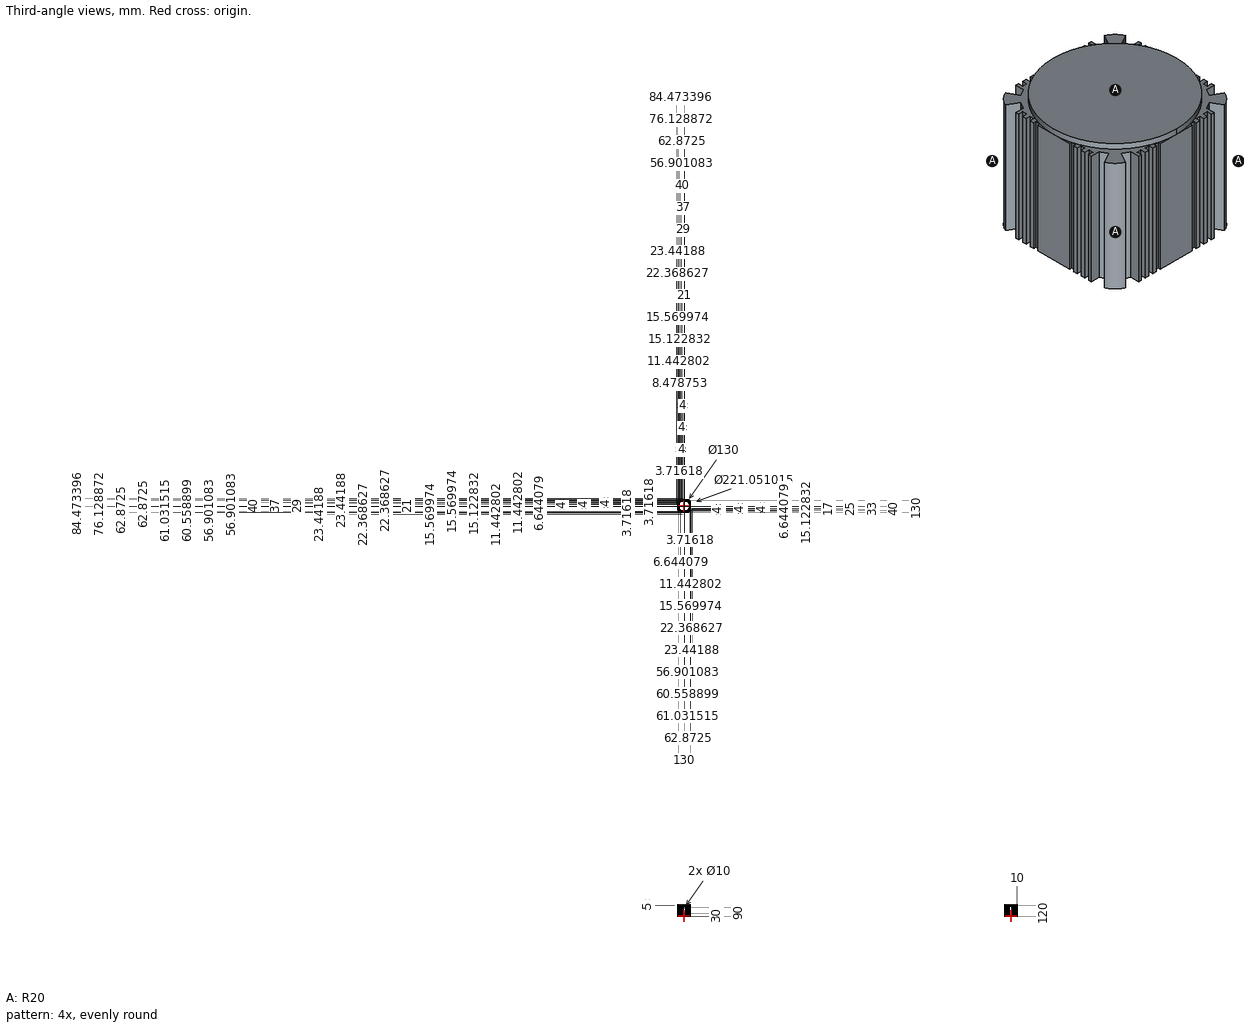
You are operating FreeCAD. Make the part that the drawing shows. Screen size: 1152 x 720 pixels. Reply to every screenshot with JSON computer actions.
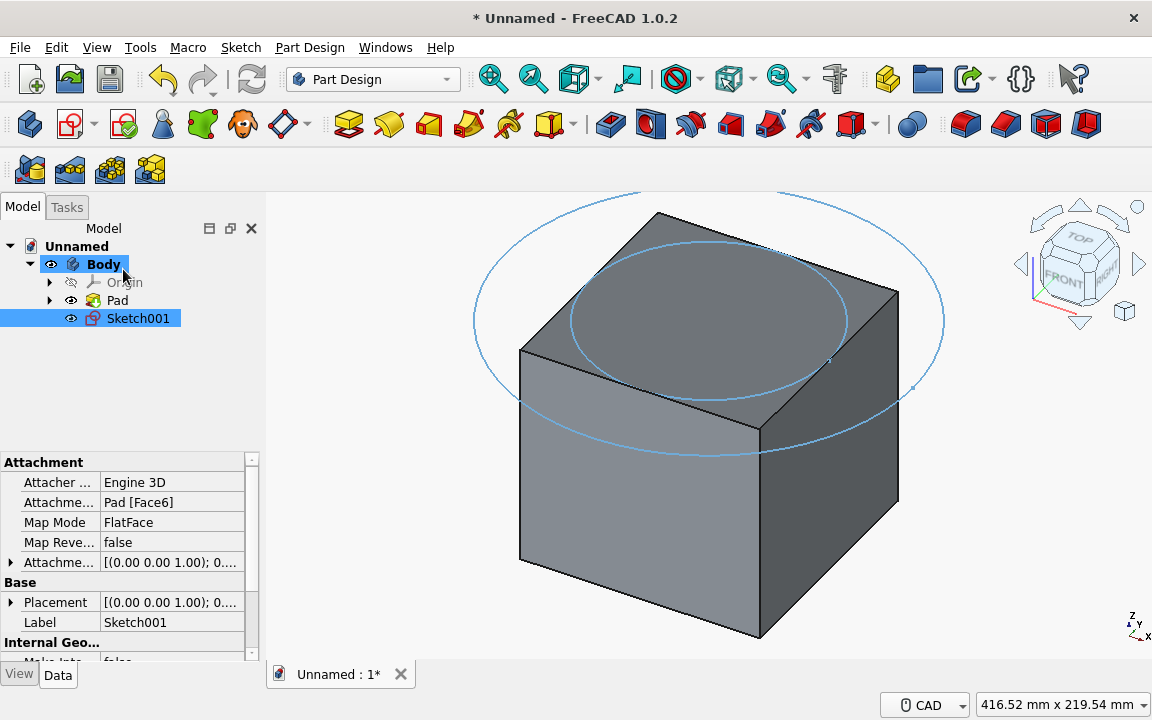
{"action": "left_click", "coordinate": [612, 124]}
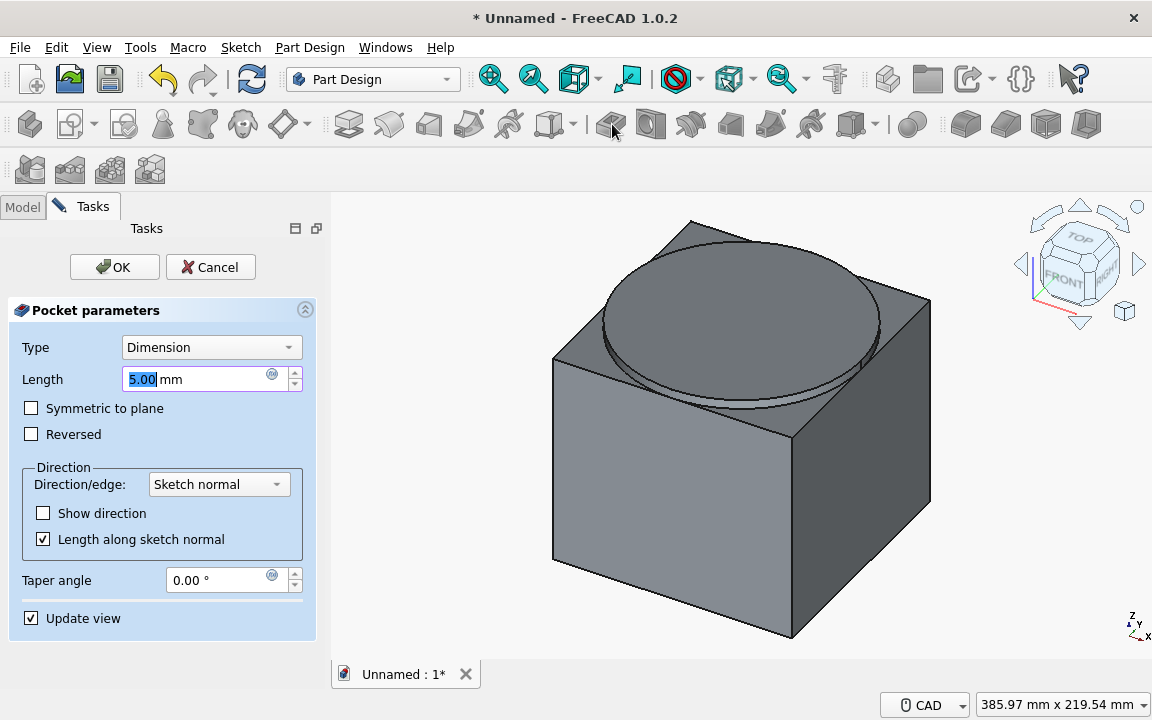
{"action": "type", "text": "5"}
{"action": "key", "text": "Tab"}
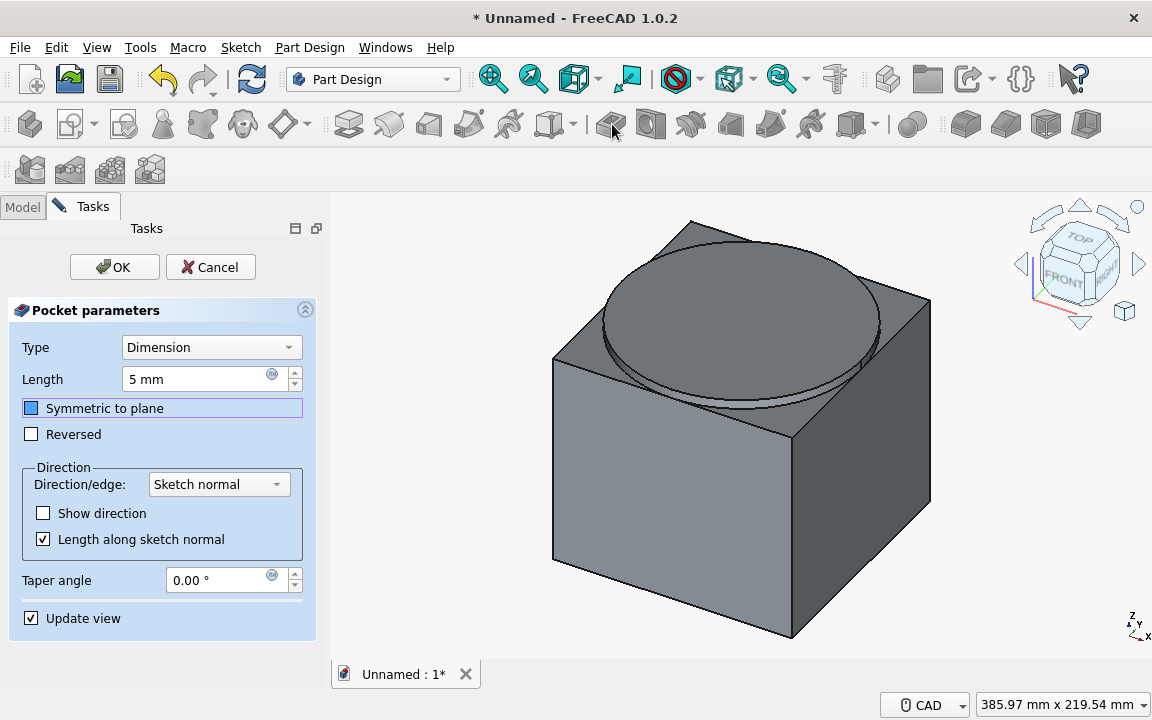
{"action": "left_click", "coordinate": [115, 267]}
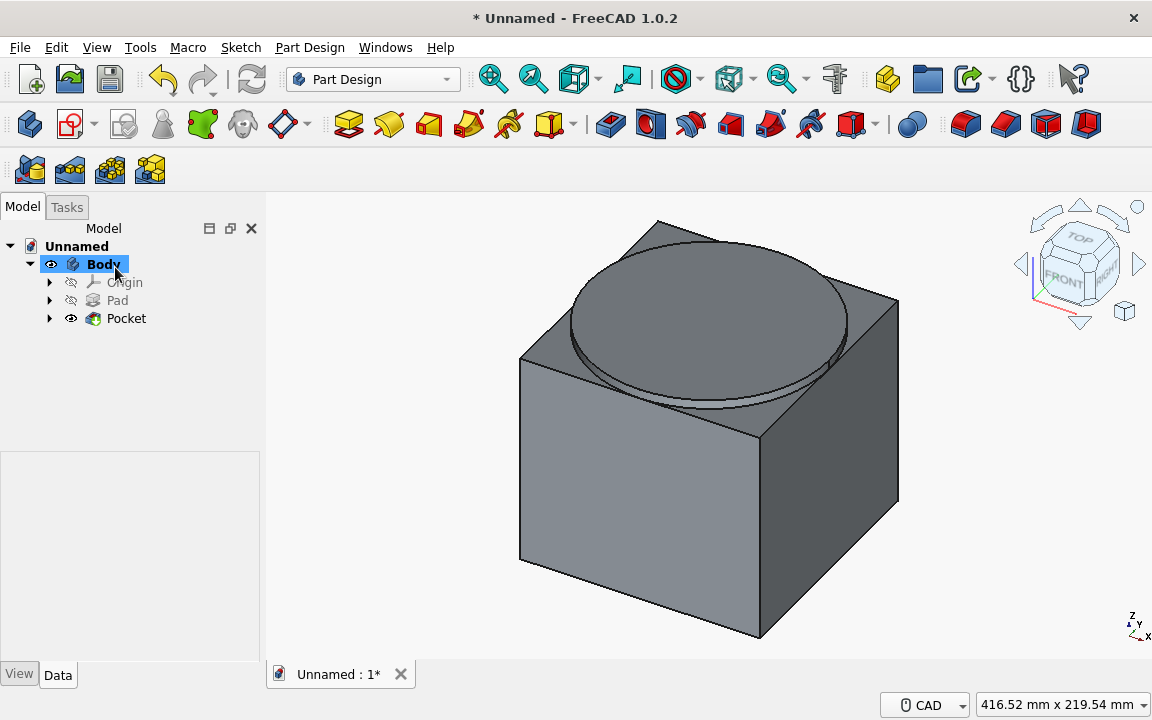
{"action": "left_click", "coordinate": [760, 537]}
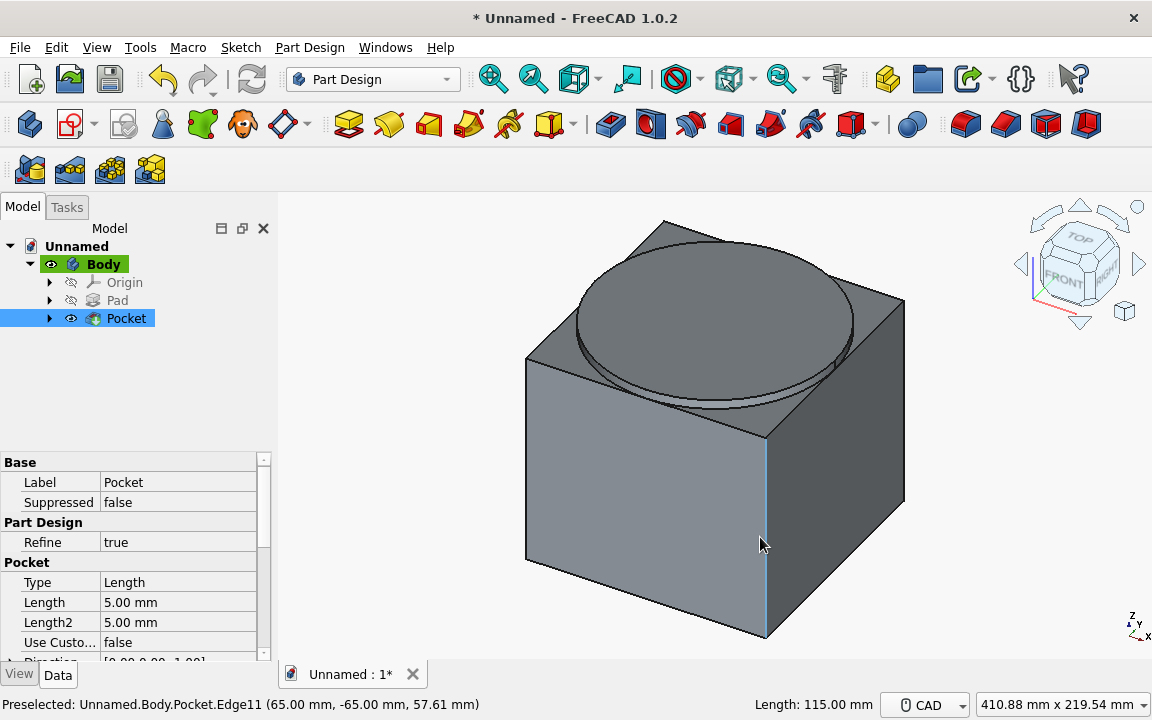
{"action": "key", "text": "0"}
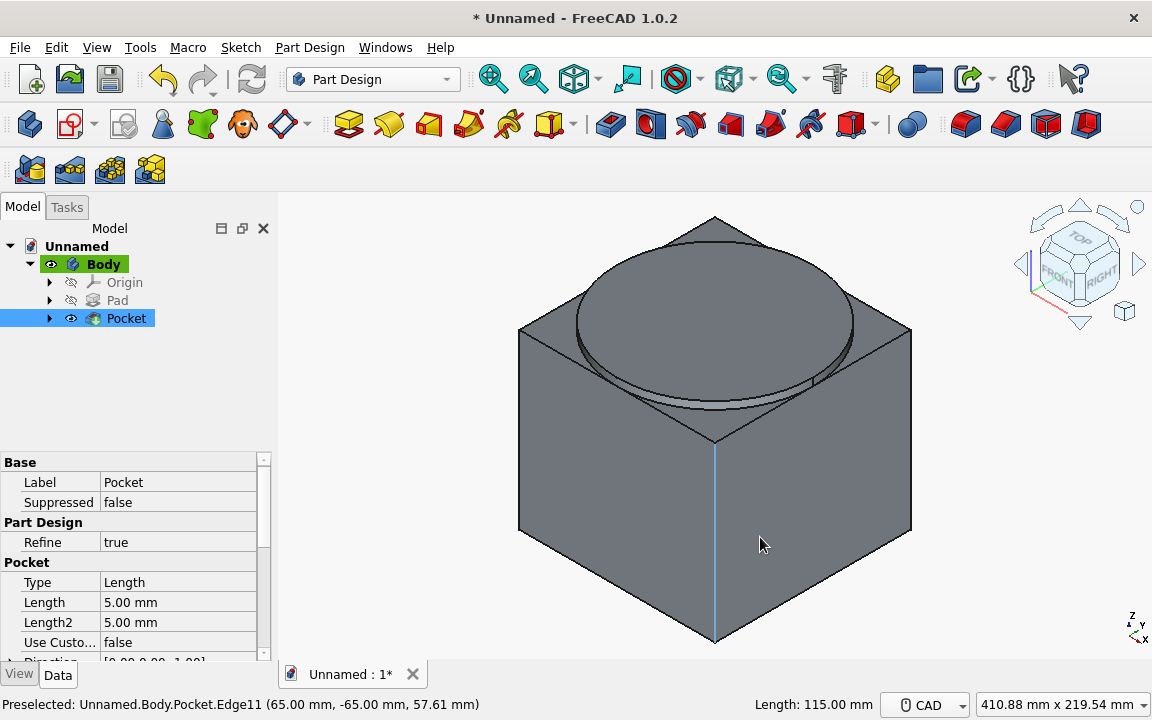
{"action": "key", "text": "2"}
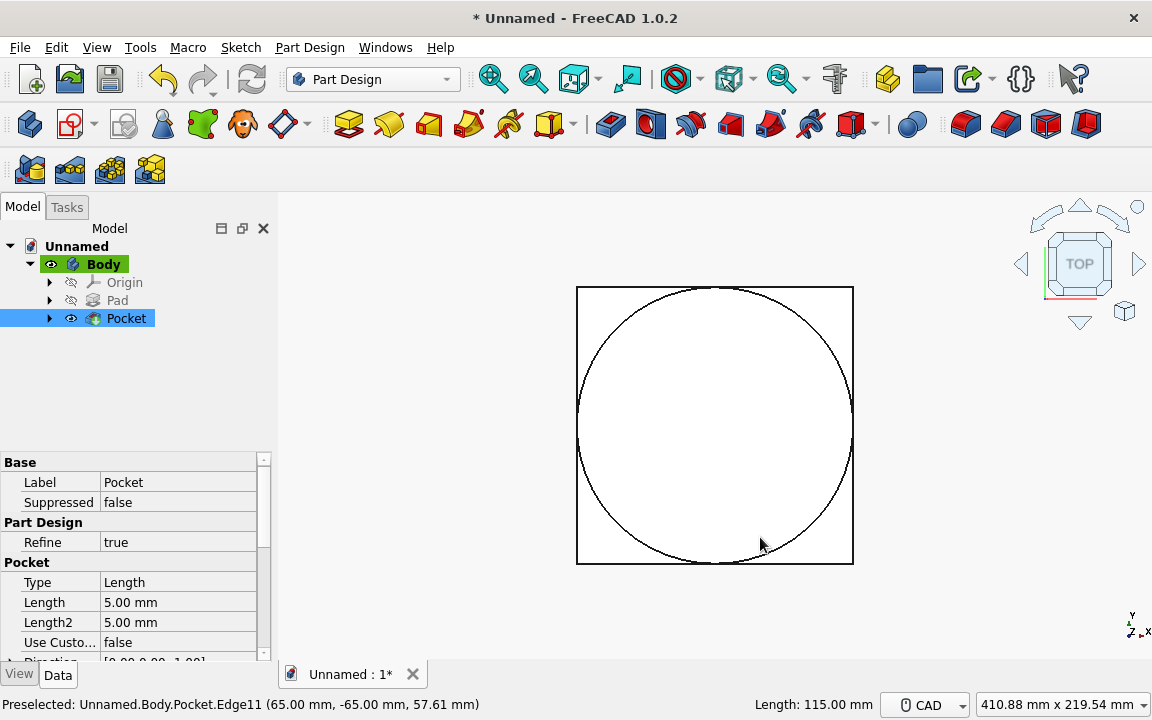
{"action": "key", "text": "1"}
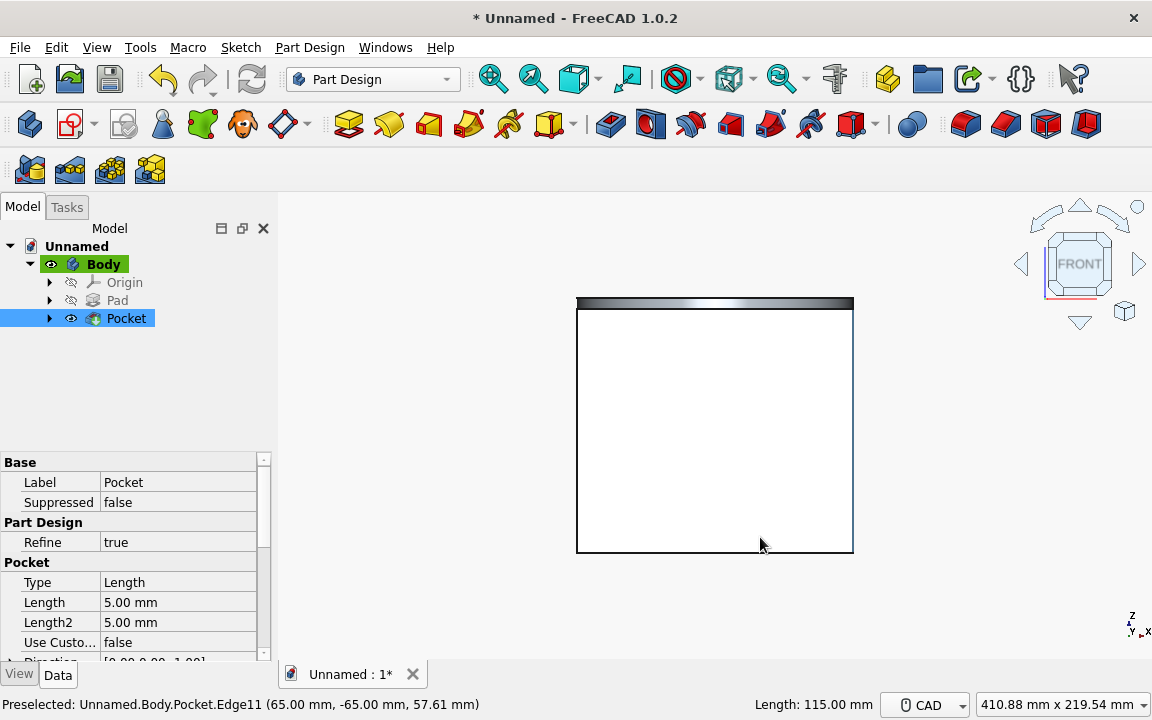
{"action": "left_click", "coordinate": [577, 430], "text": "ctrl"}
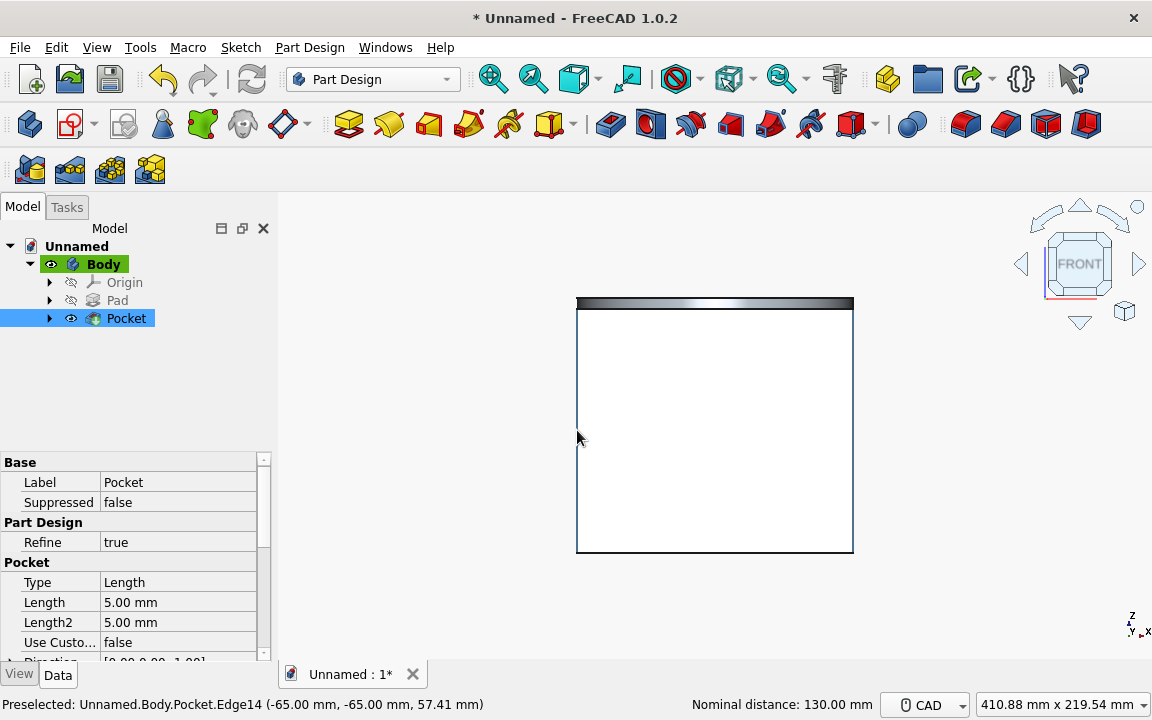
{"action": "key", "text": "3"}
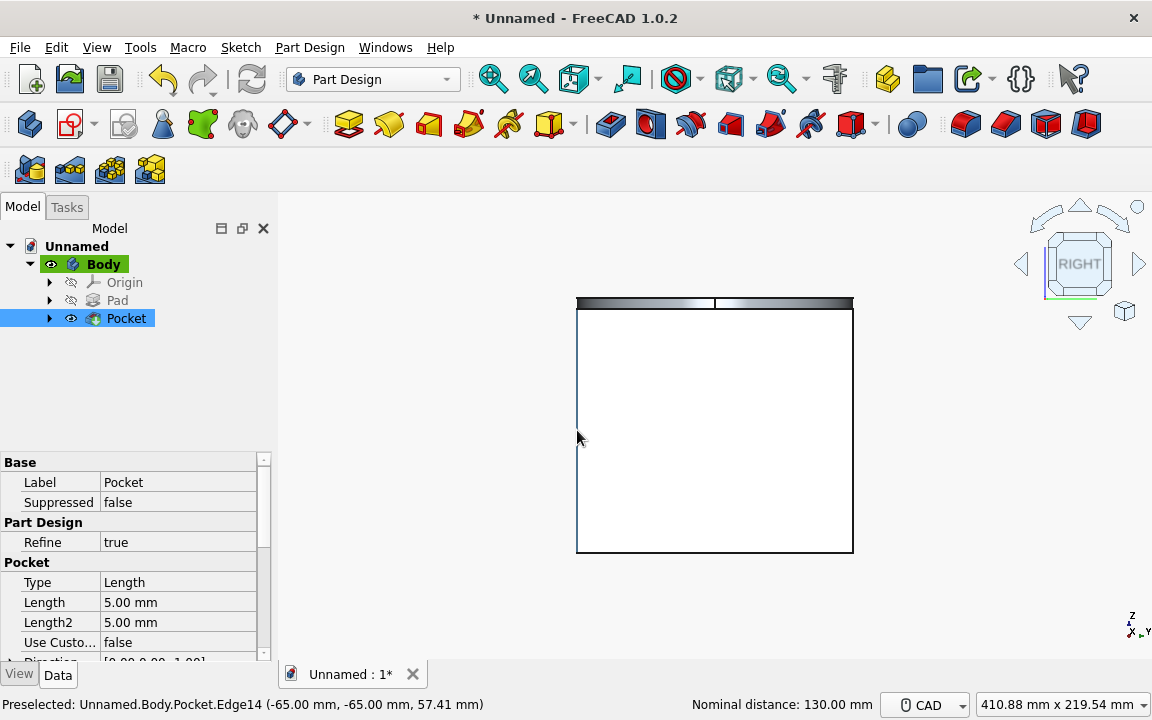
{"action": "left_click", "coordinate": [853, 430], "text": "ctrl"}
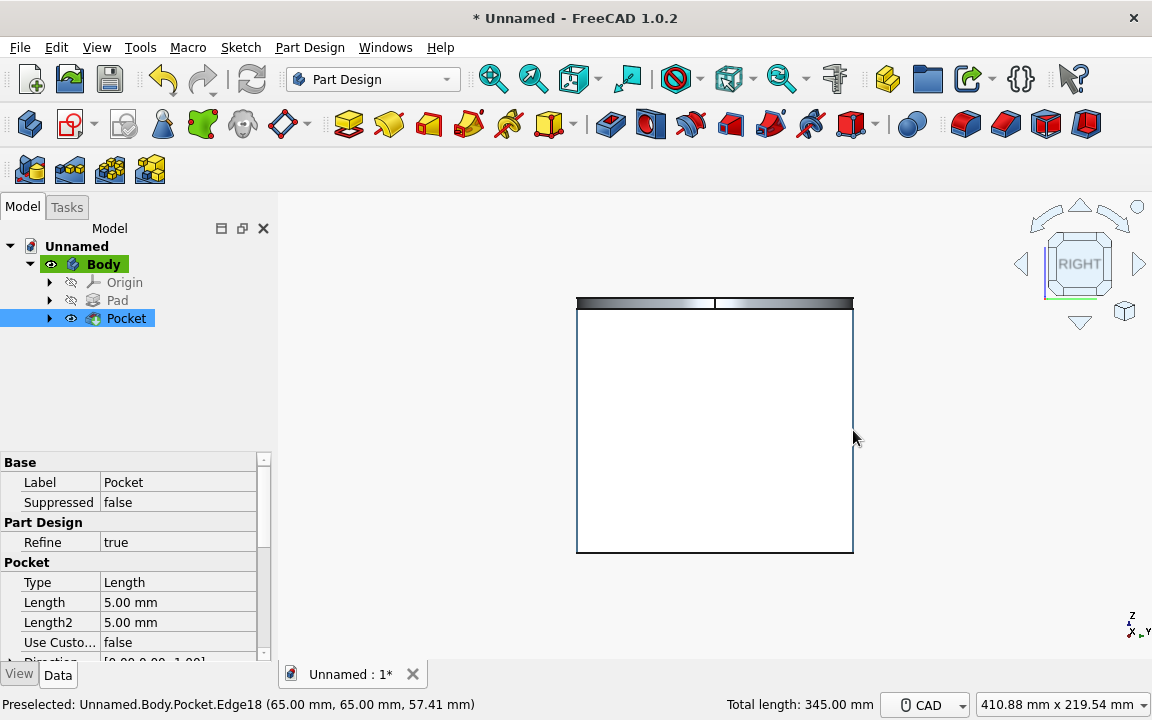
{"action": "key", "text": "5"}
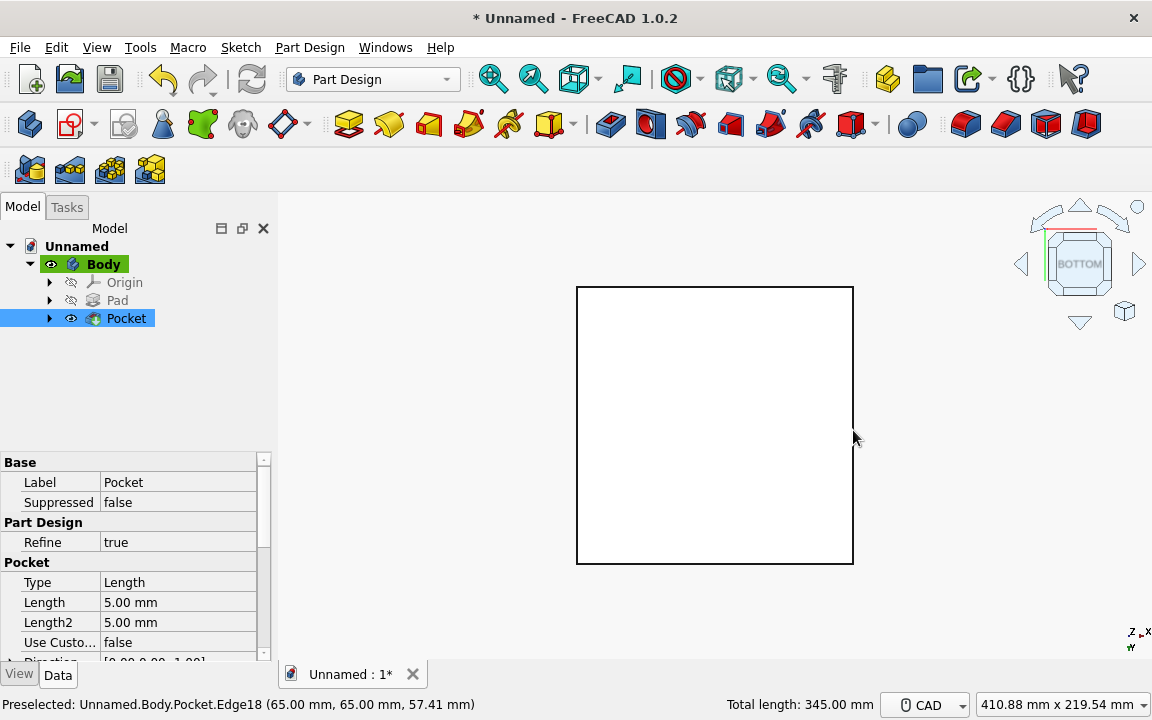
{"action": "key", "text": "4"}